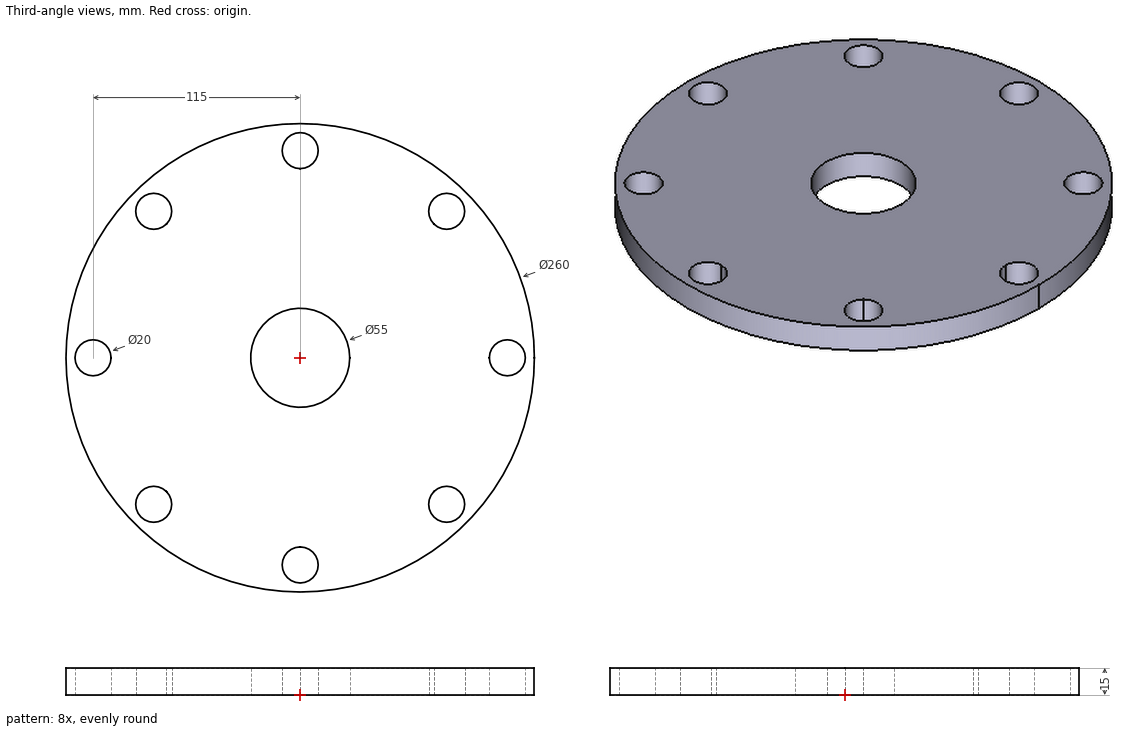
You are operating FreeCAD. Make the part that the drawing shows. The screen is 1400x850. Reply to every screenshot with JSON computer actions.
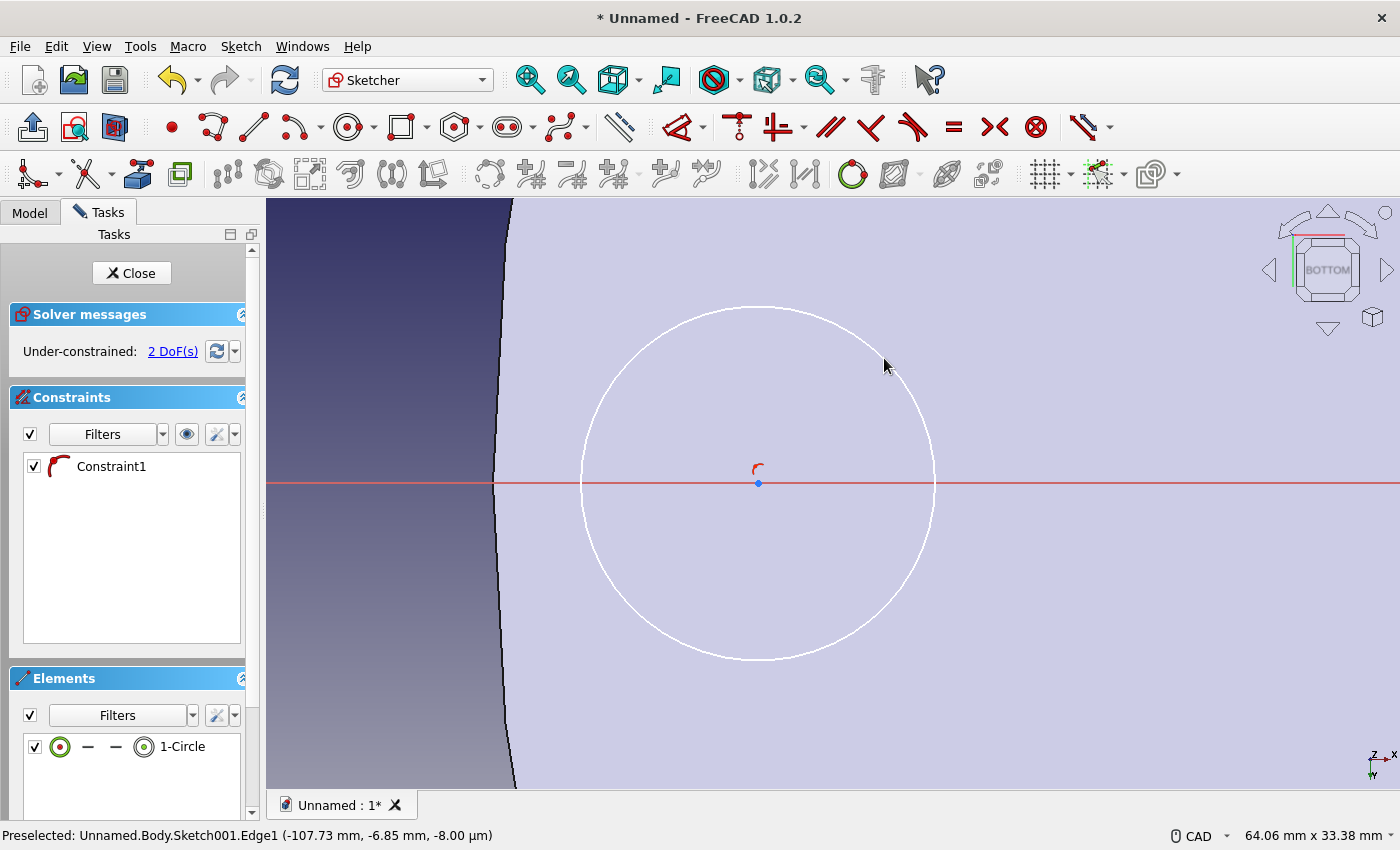
{"action": "left_click", "coordinate": [676, 128]}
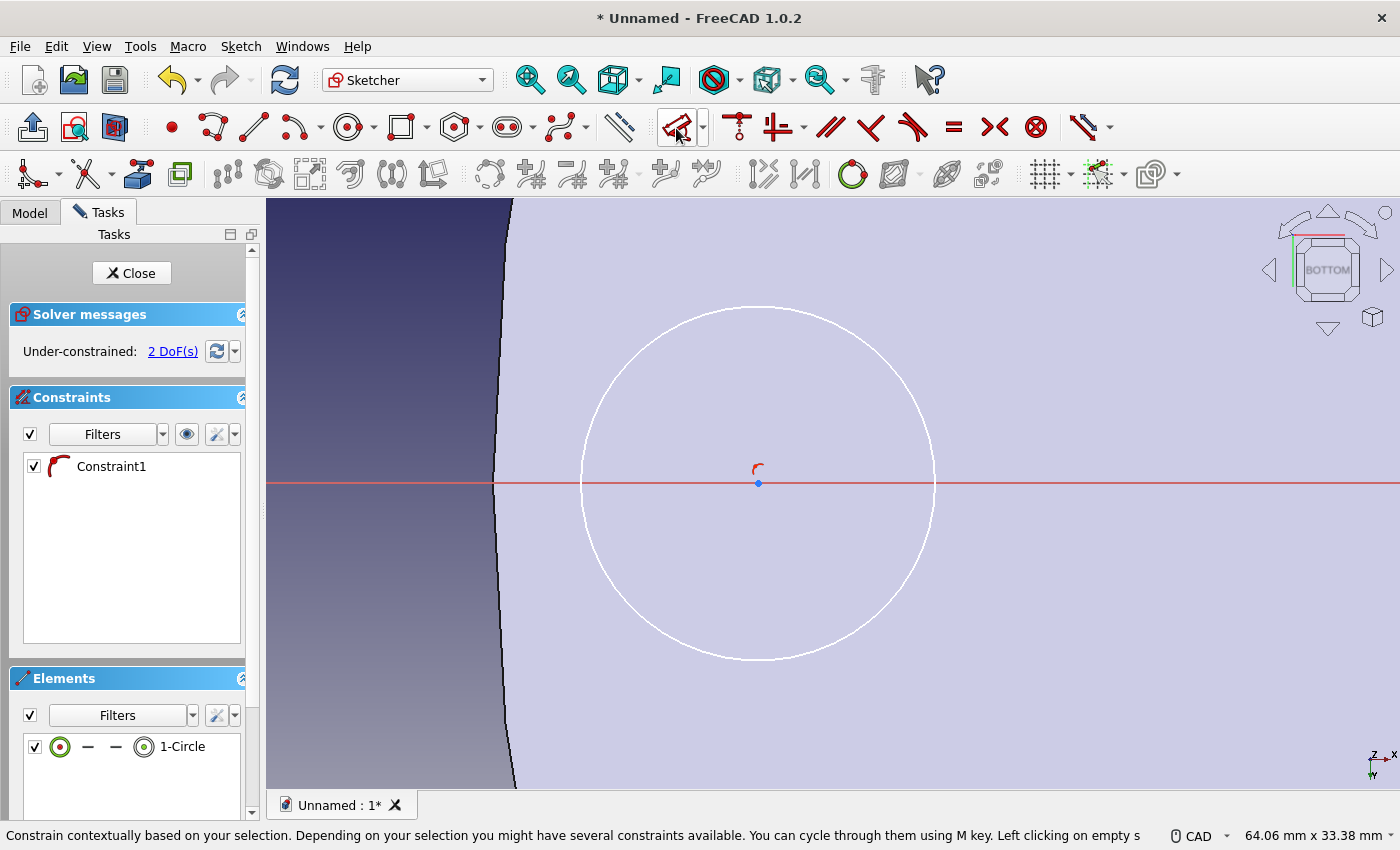
{"action": "left_click", "coordinate": [883, 358]}
{"action": "left_click", "coordinate": [906, 335]}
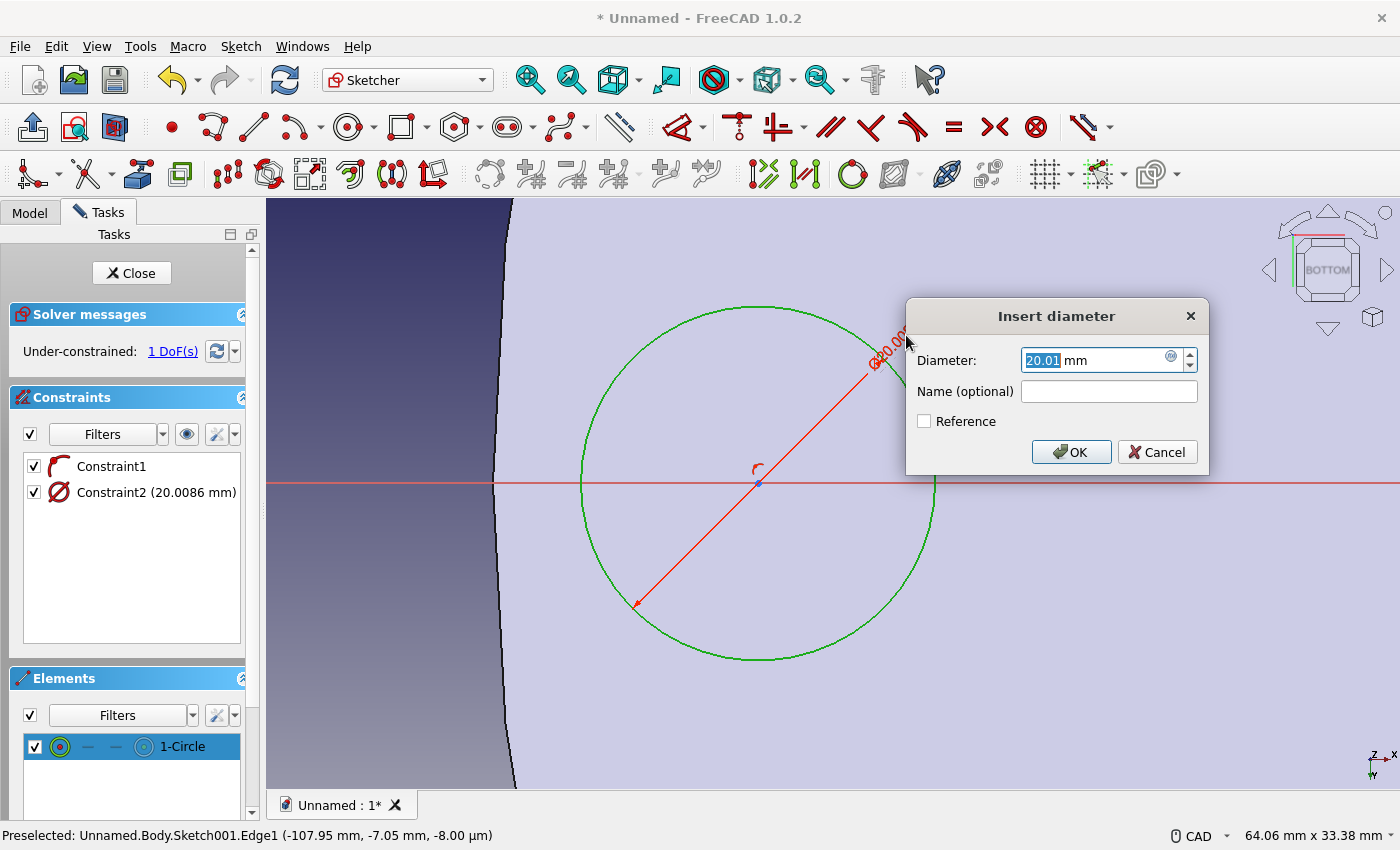
{"action": "type", "text": "20"}
{"action": "key", "text": "Return"}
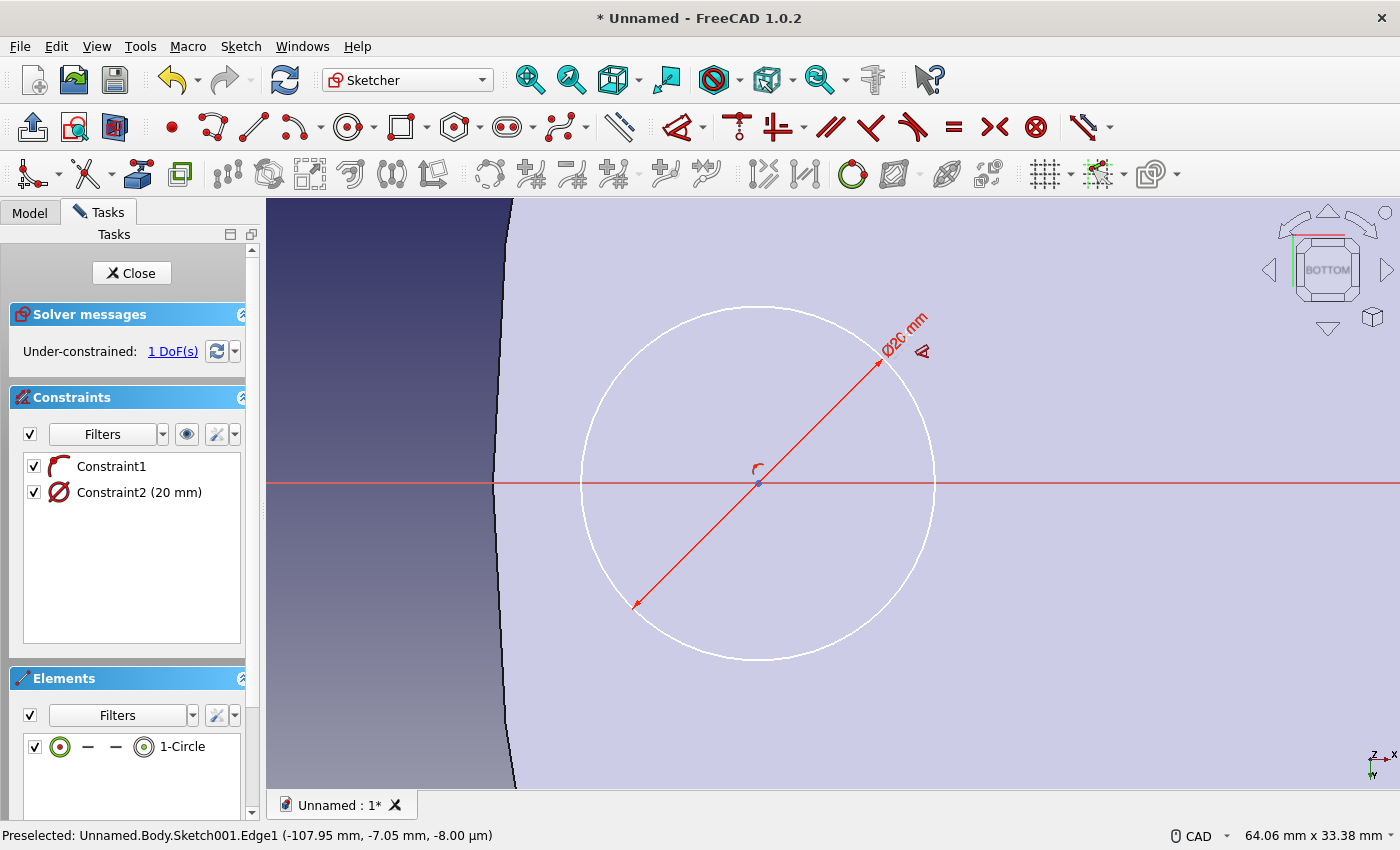
{"action": "left_click", "coordinate": [758, 483]}
{"action": "left_click", "coordinate": [997, 517]}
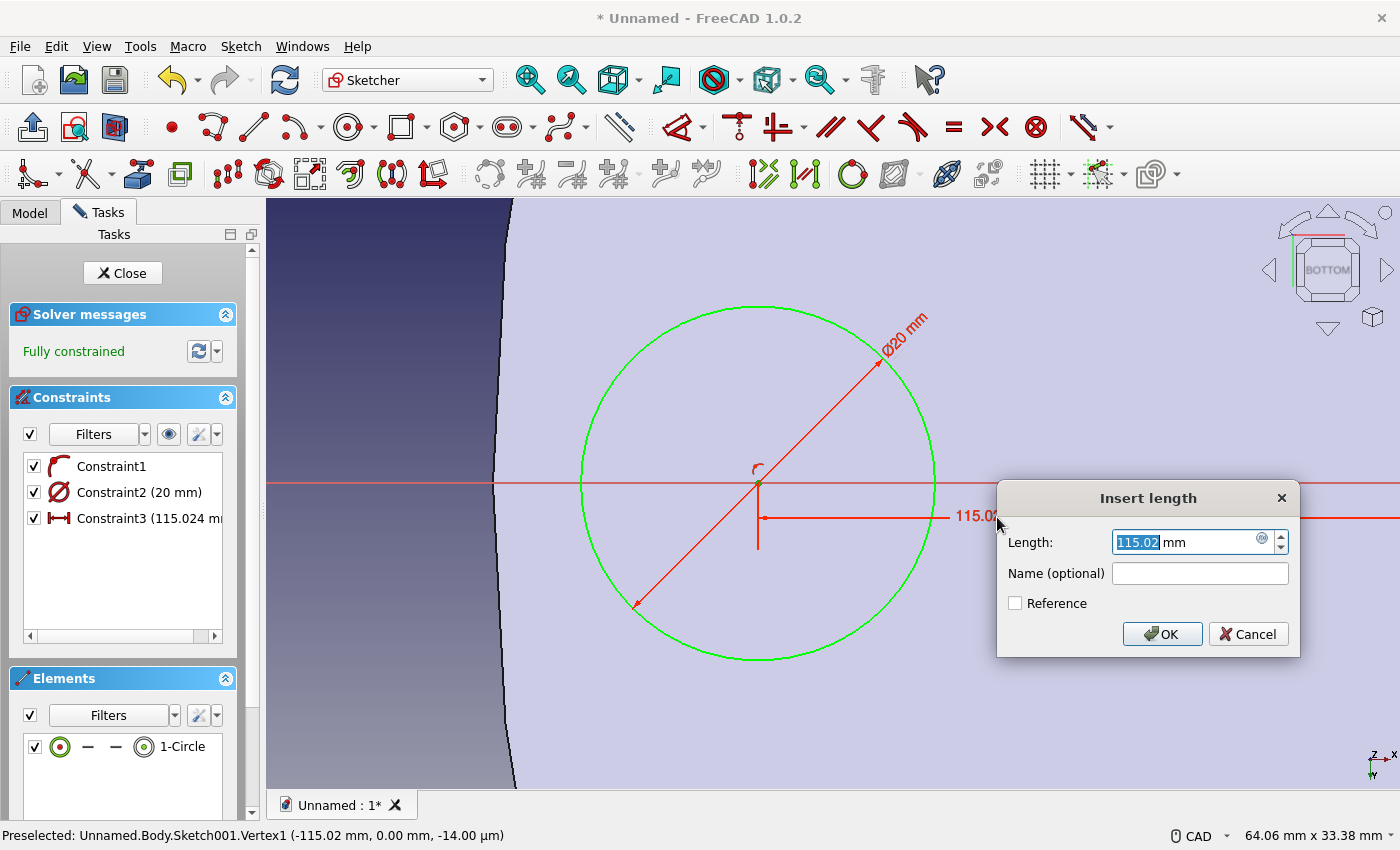
{"action": "type", "text": "115"}
{"action": "key", "text": "Return"}
{"action": "key", "text": "Escape"}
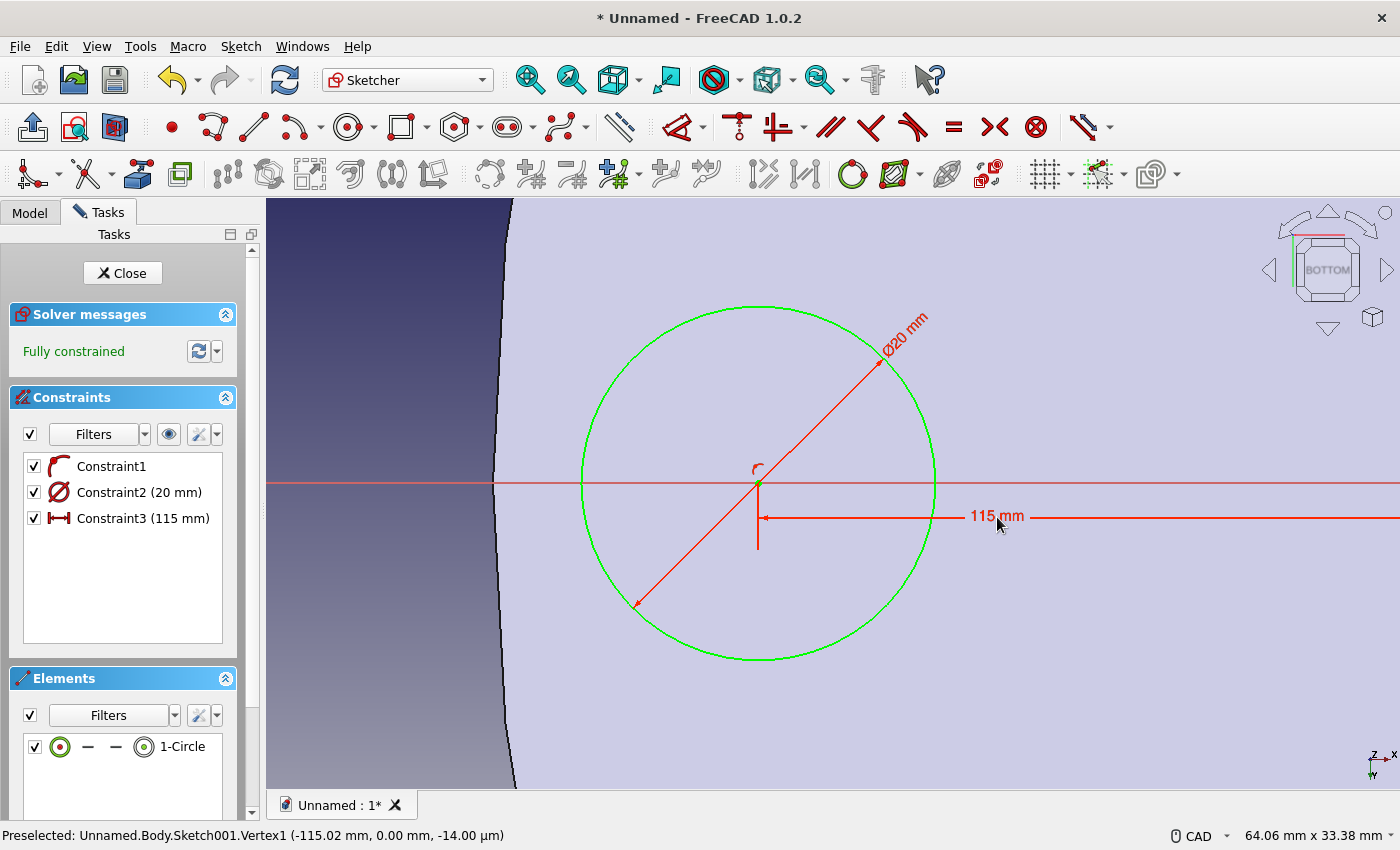
{"action": "left_click", "coordinate": [123, 273]}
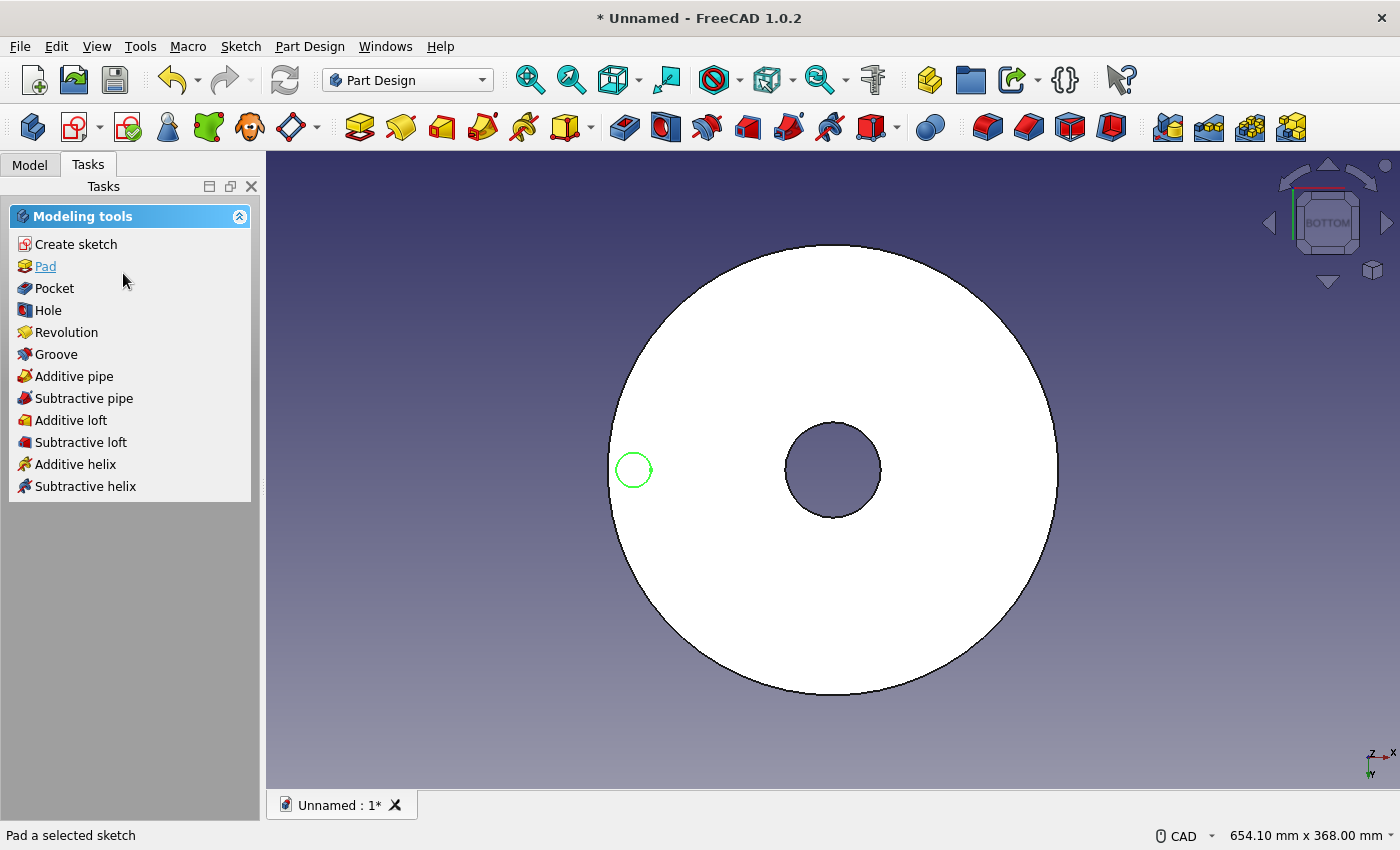
{"action": "left_click", "coordinate": [625, 128]}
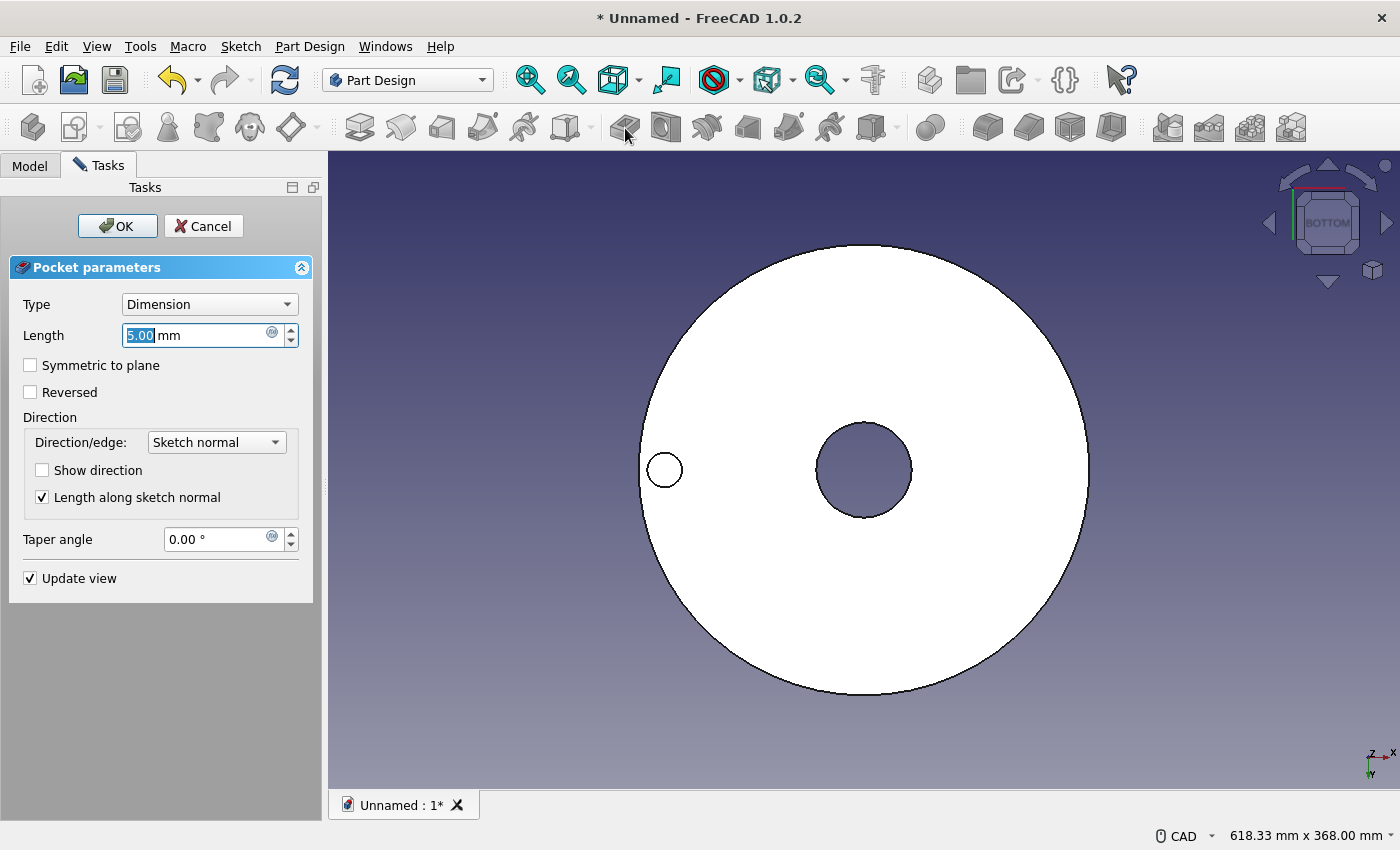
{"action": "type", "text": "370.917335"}
{"action": "key", "text": "Tab"}